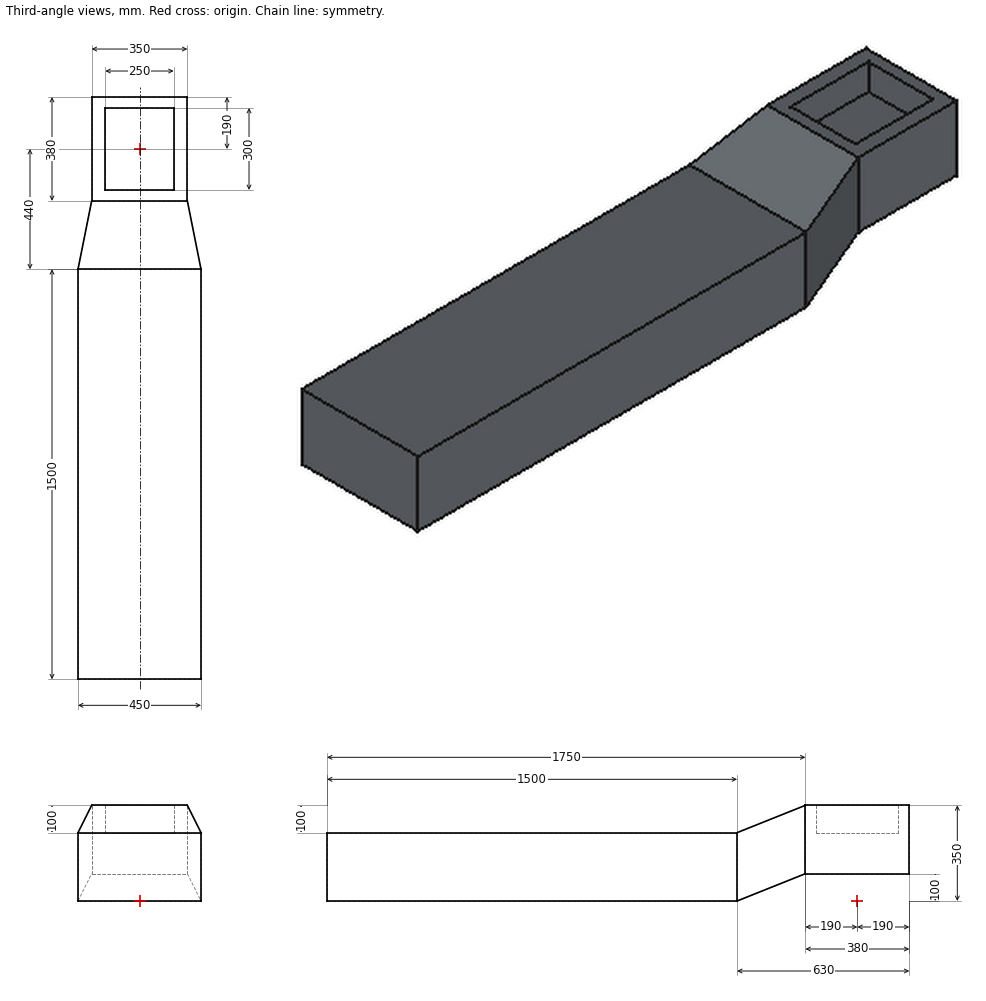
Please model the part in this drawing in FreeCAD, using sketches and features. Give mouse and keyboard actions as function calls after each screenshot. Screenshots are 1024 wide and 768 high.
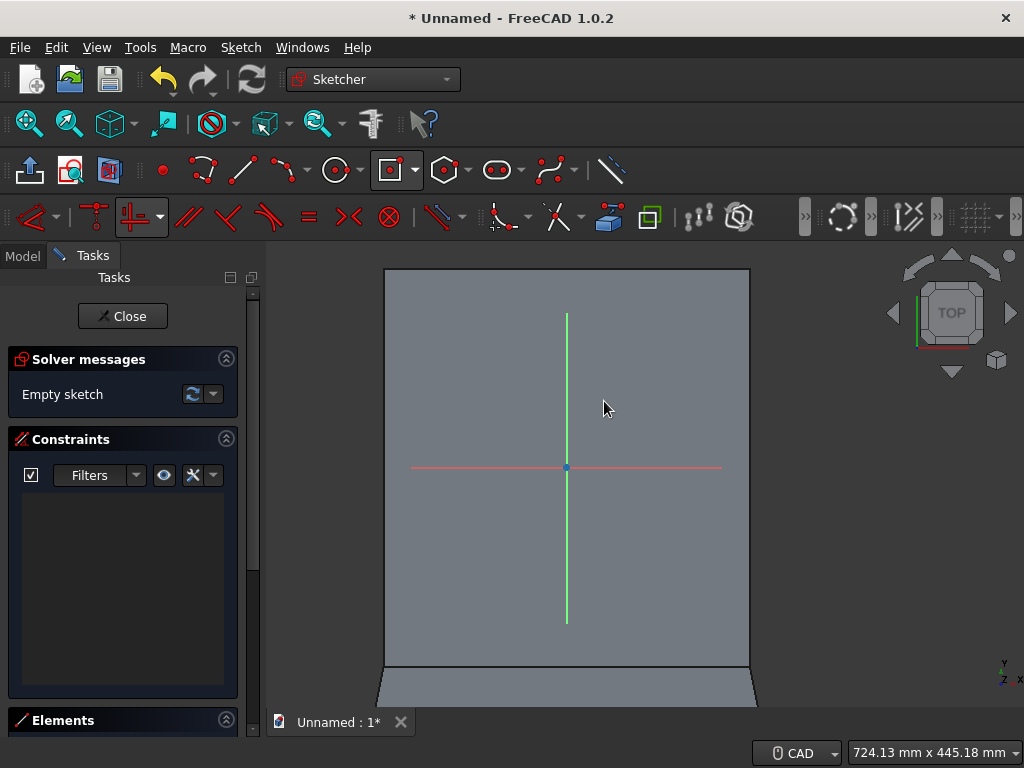
click(390, 170)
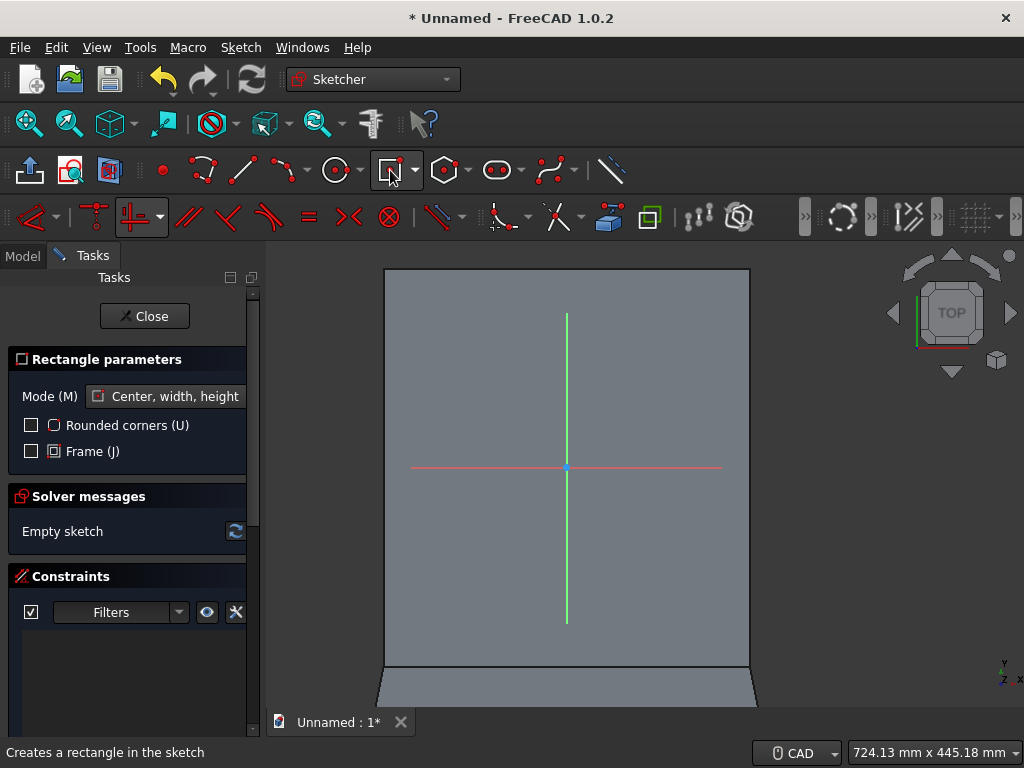
click(567, 468)
click(698, 311)
key(Escape)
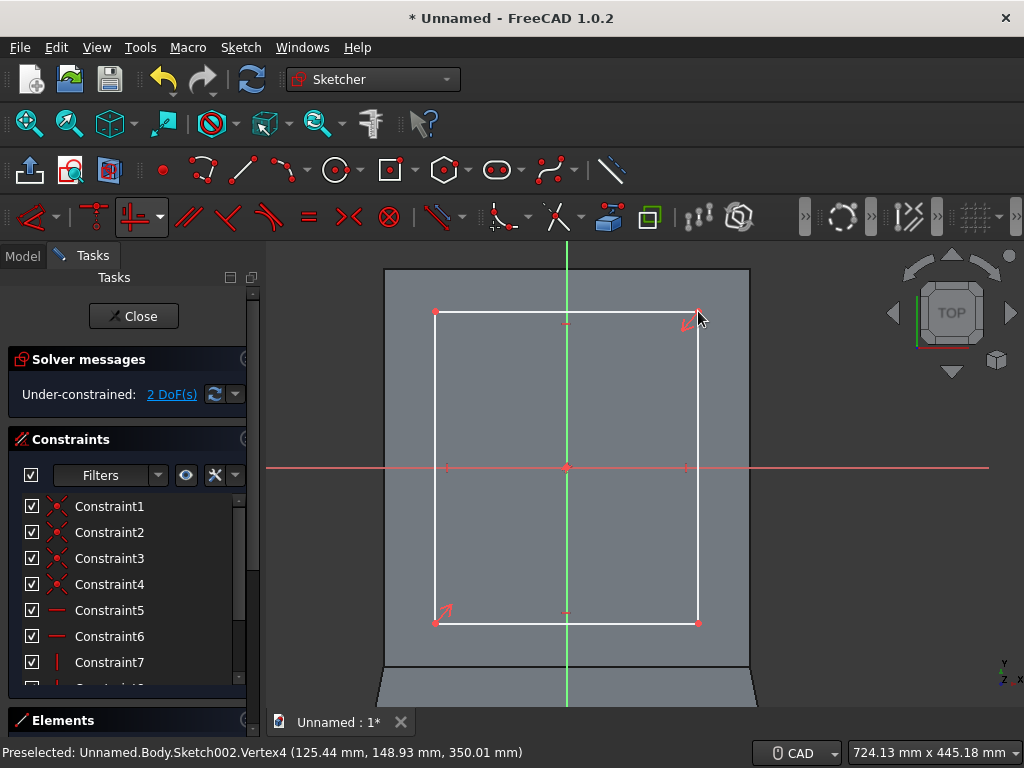
click(32, 218)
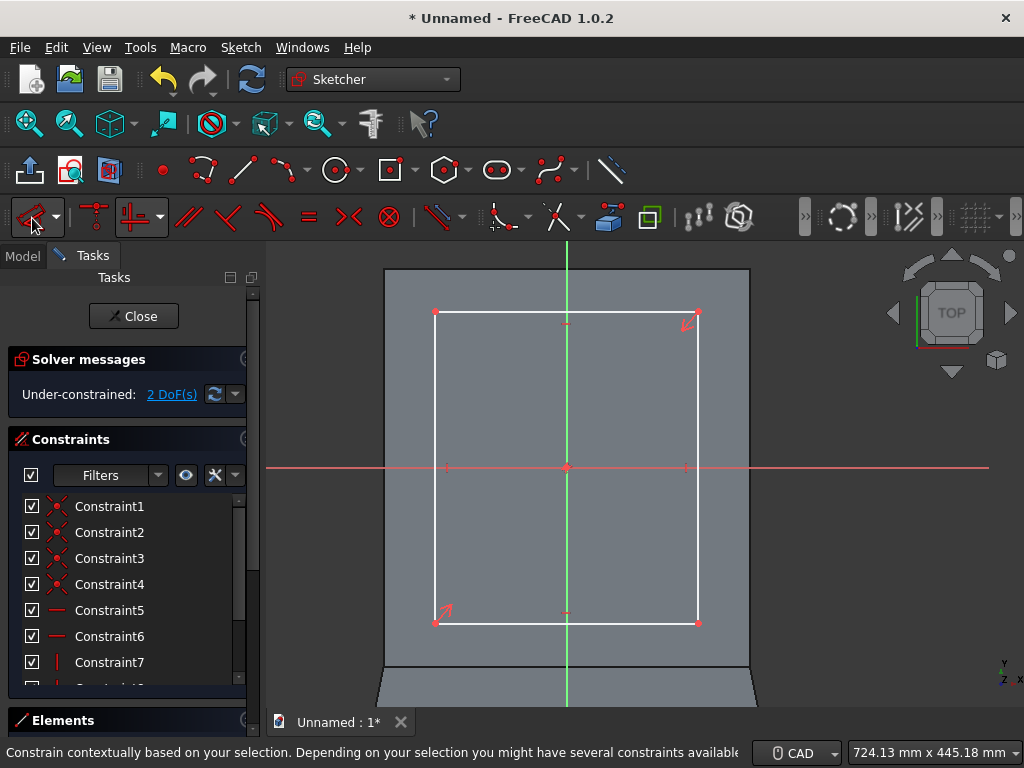
click(514, 624)
click(506, 658)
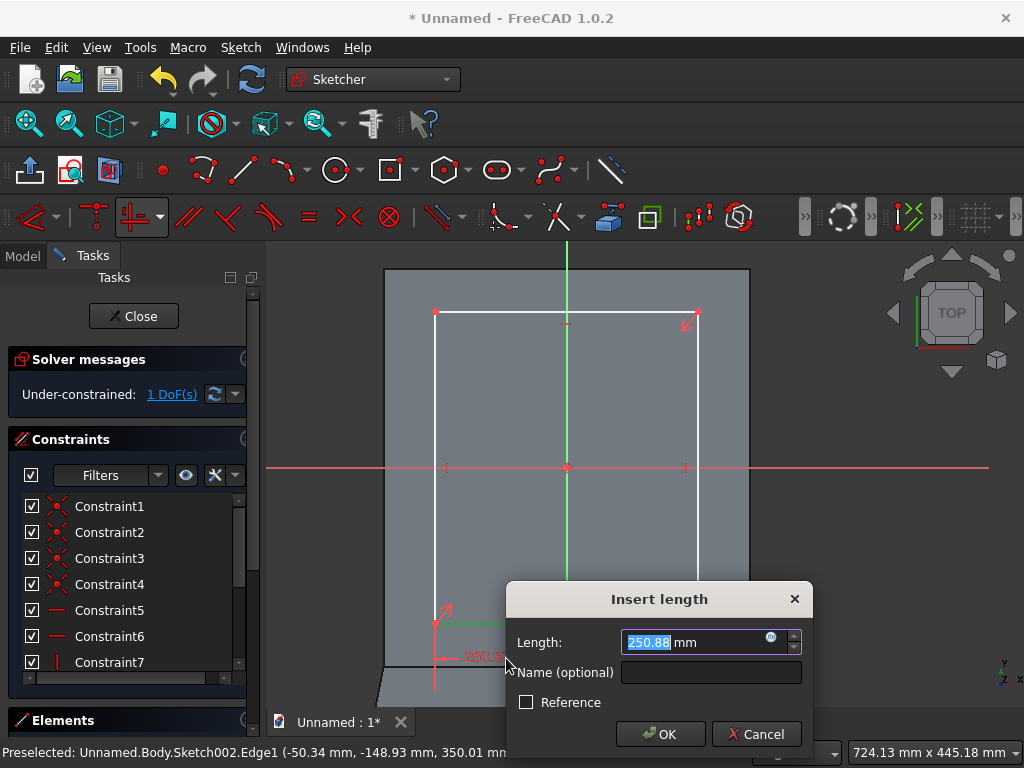
text(250)
key(Return)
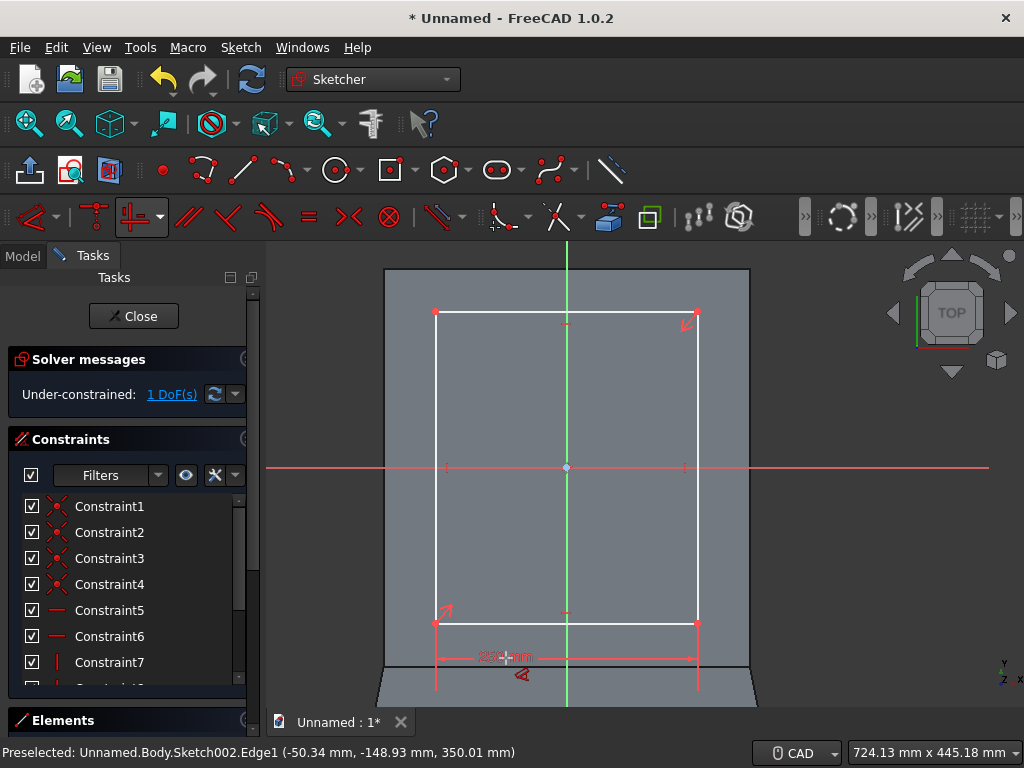
click(698, 530)
click(732, 396)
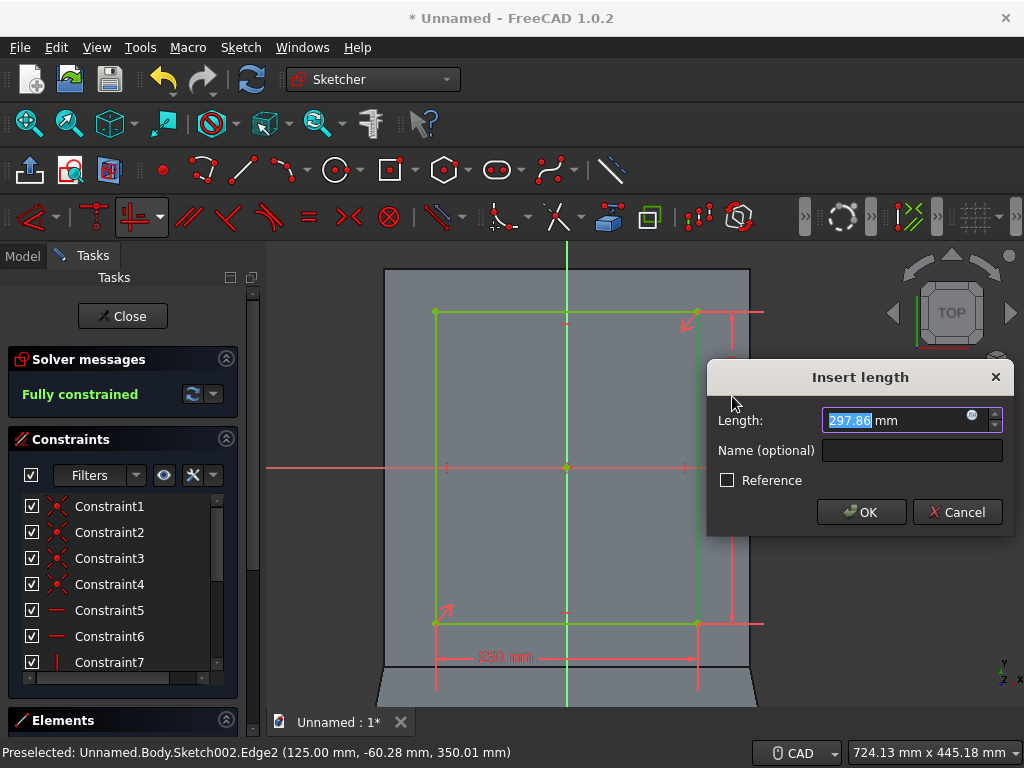
text(300)
key(Return)
key(Escape)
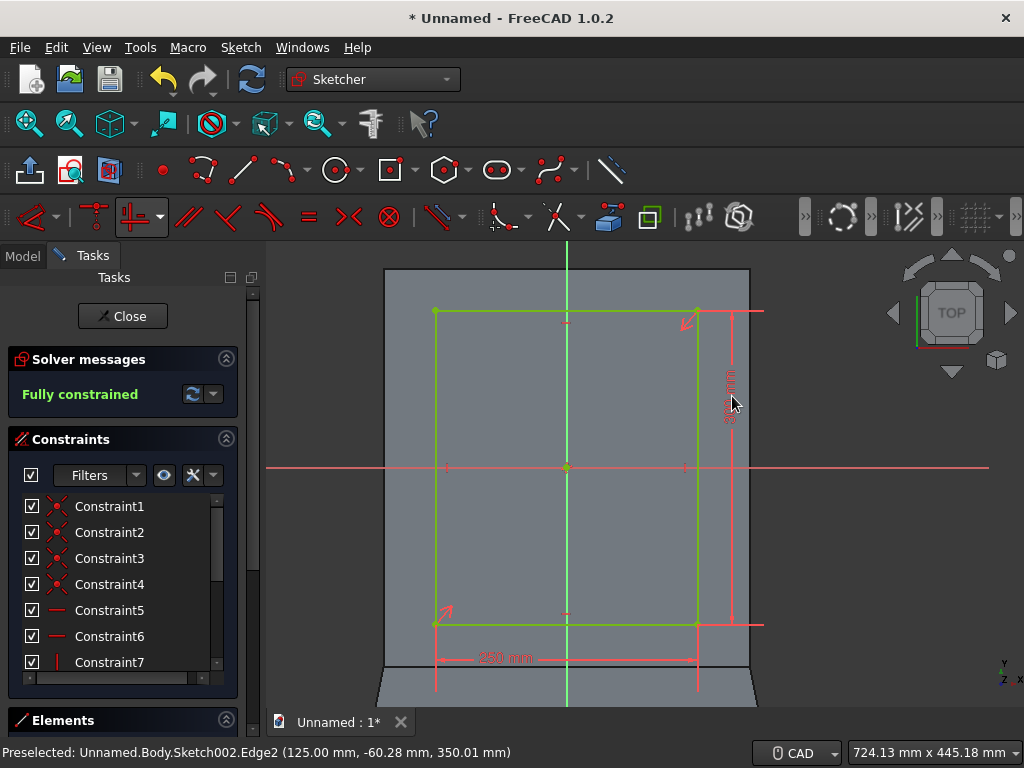
click(123, 316)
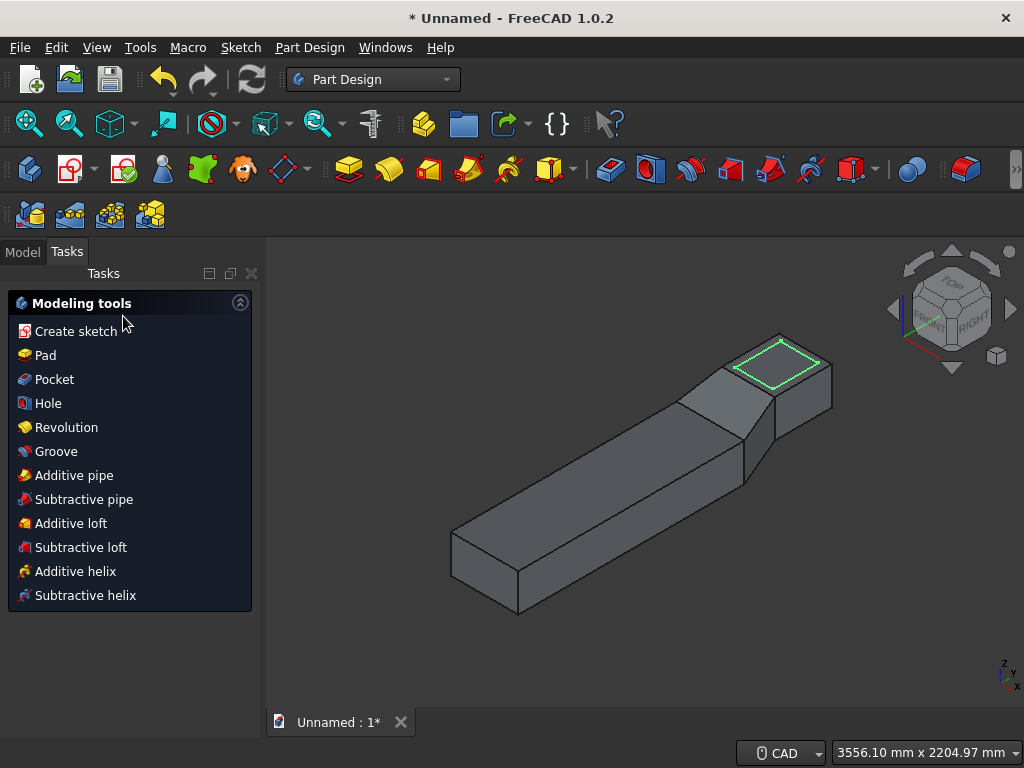
click(612, 170)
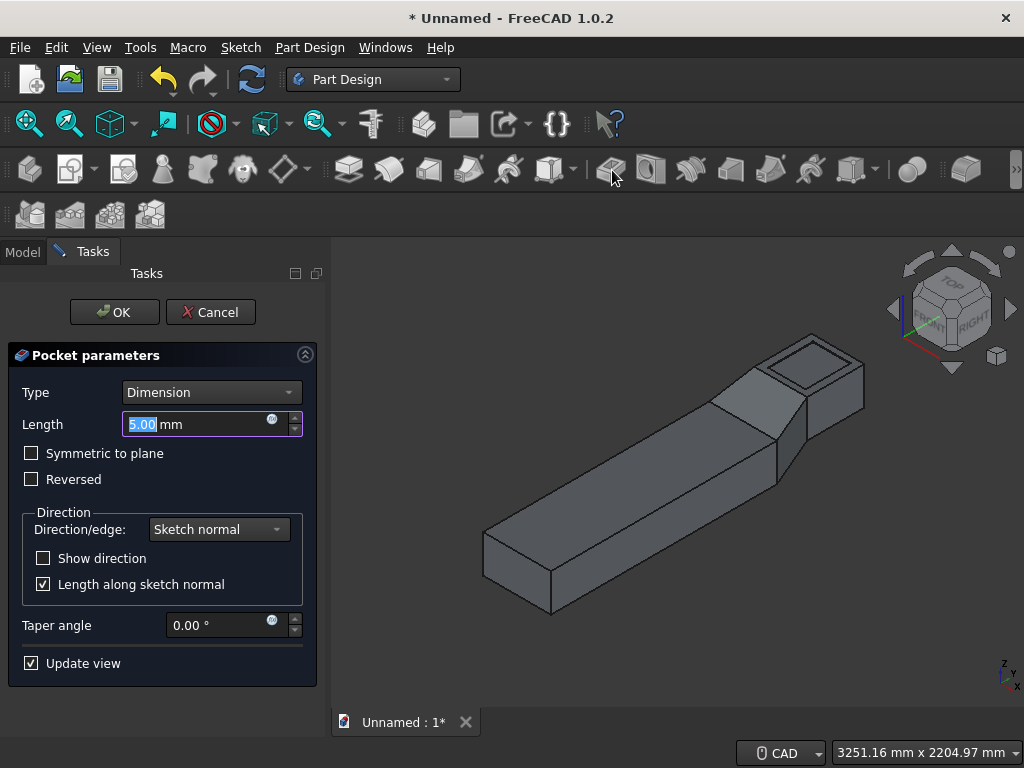
text(100)
key(Tab)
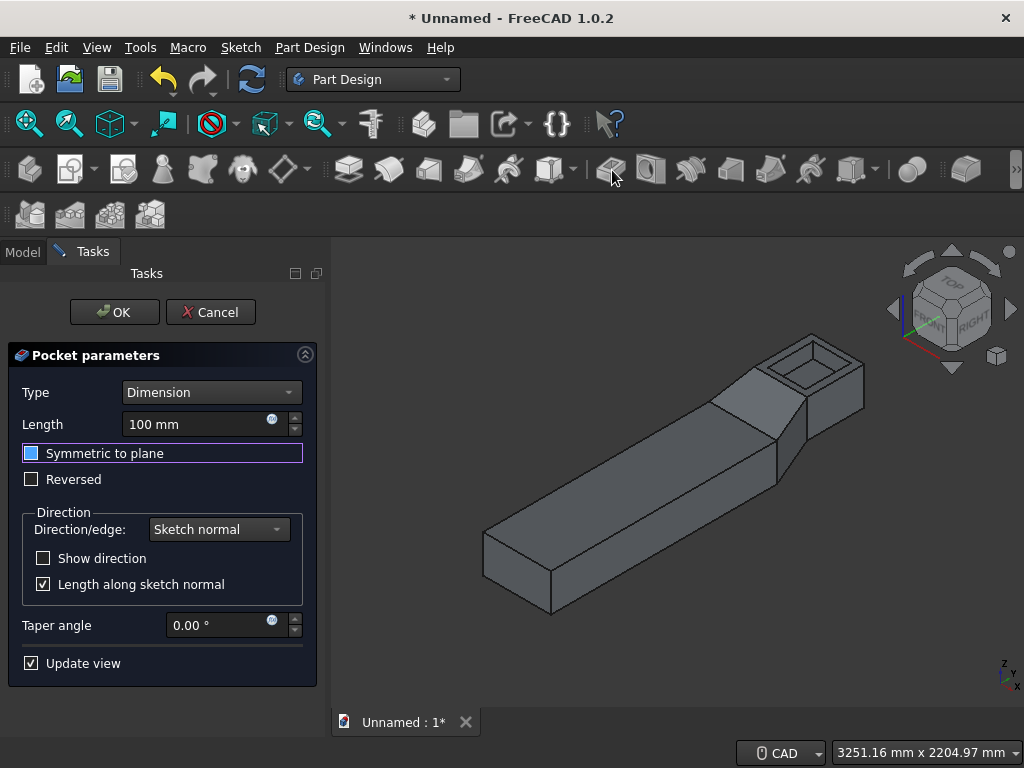
click(115, 312)